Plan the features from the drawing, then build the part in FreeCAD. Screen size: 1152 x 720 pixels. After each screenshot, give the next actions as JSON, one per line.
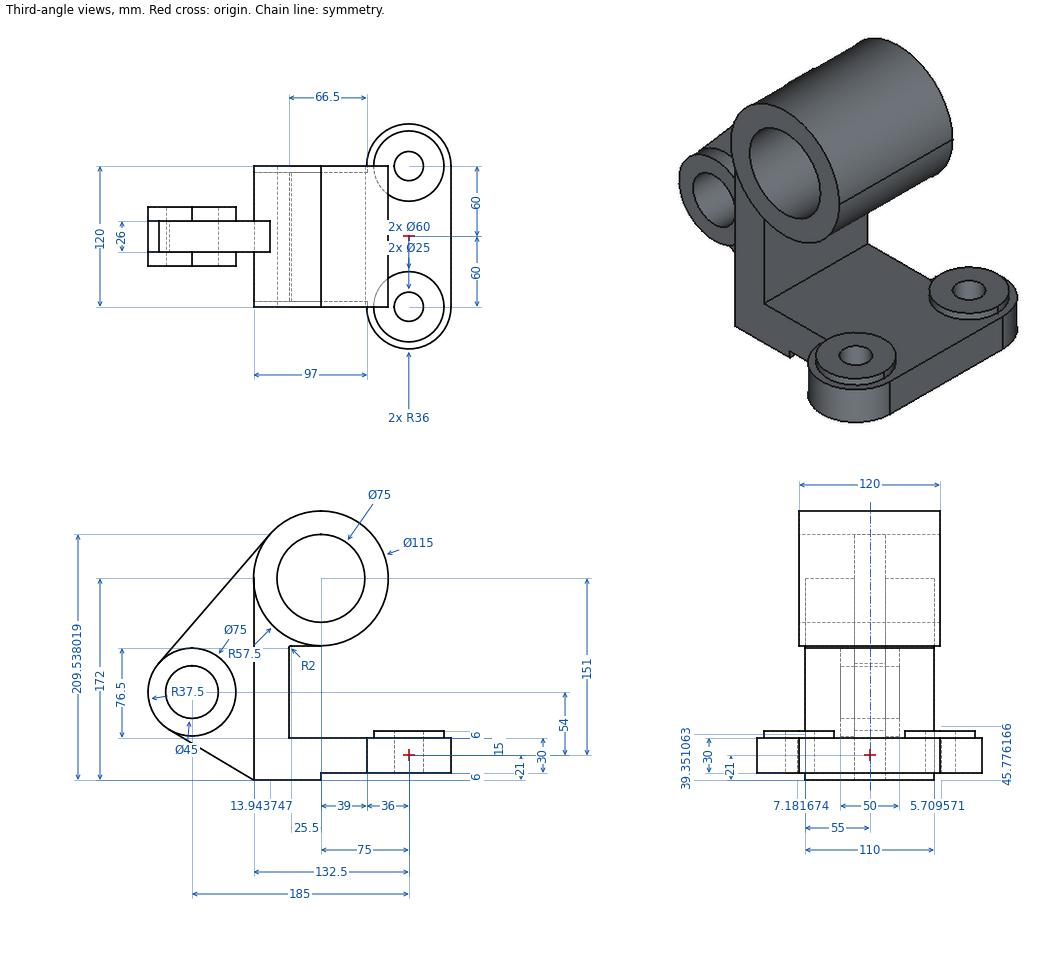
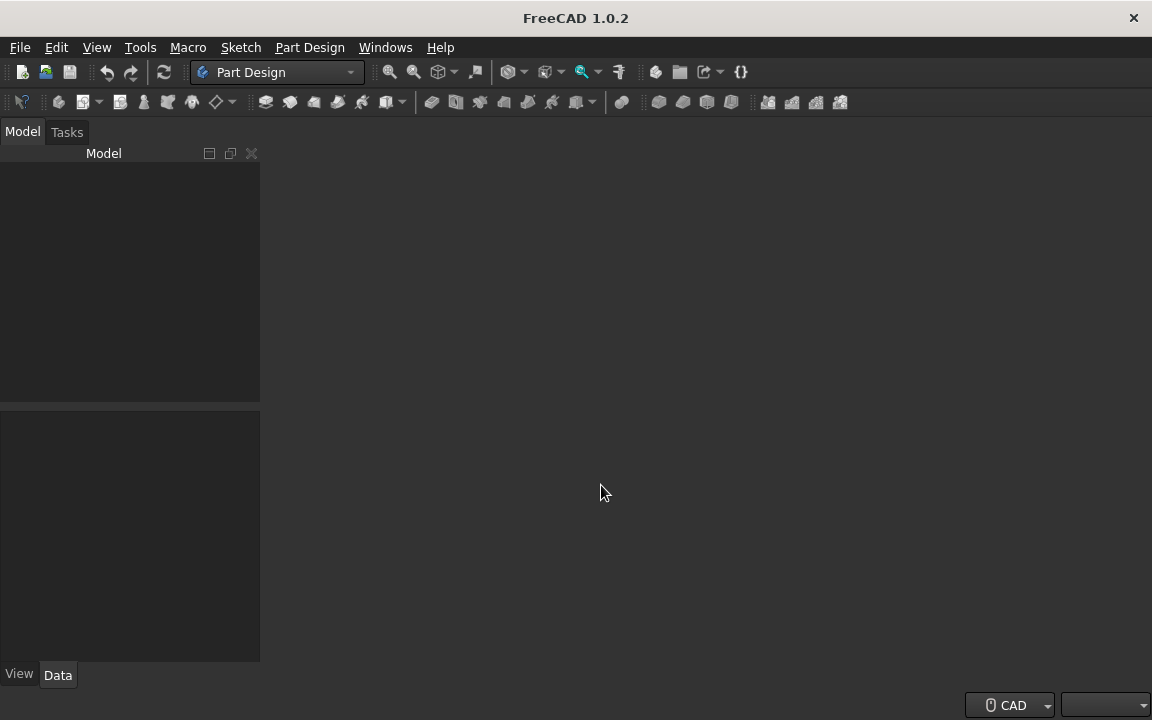
{"action": "left_click", "coordinate": [22, 72]}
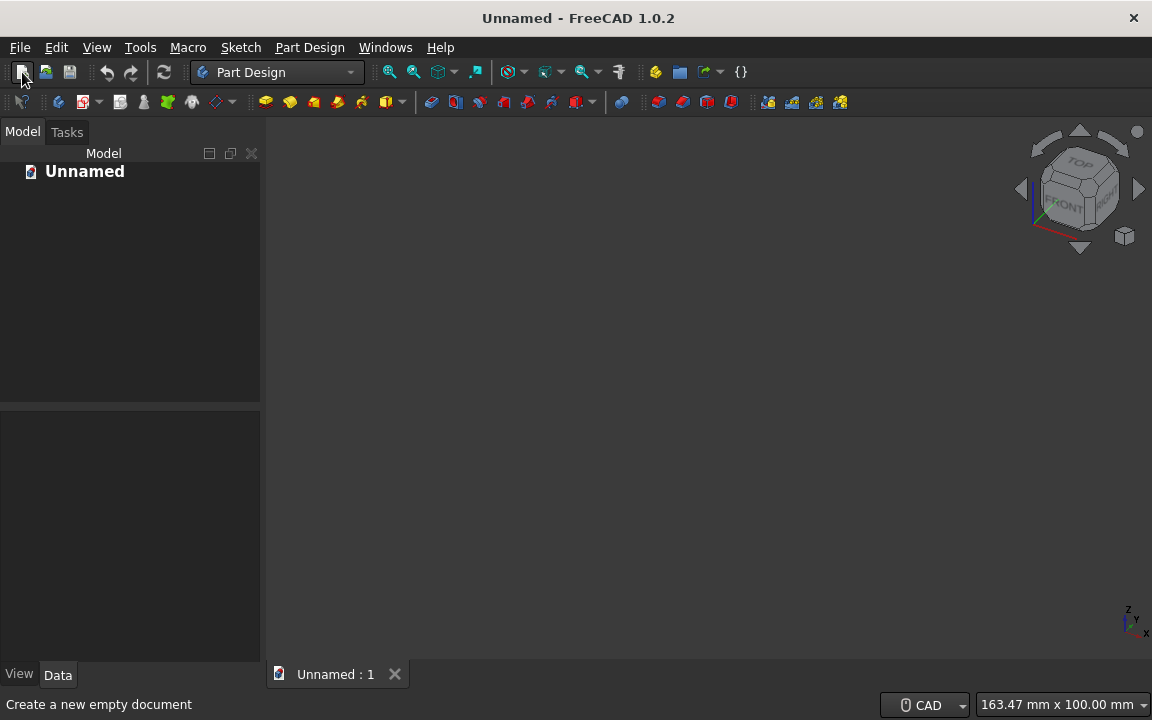
{"action": "left_click", "coordinate": [84, 102]}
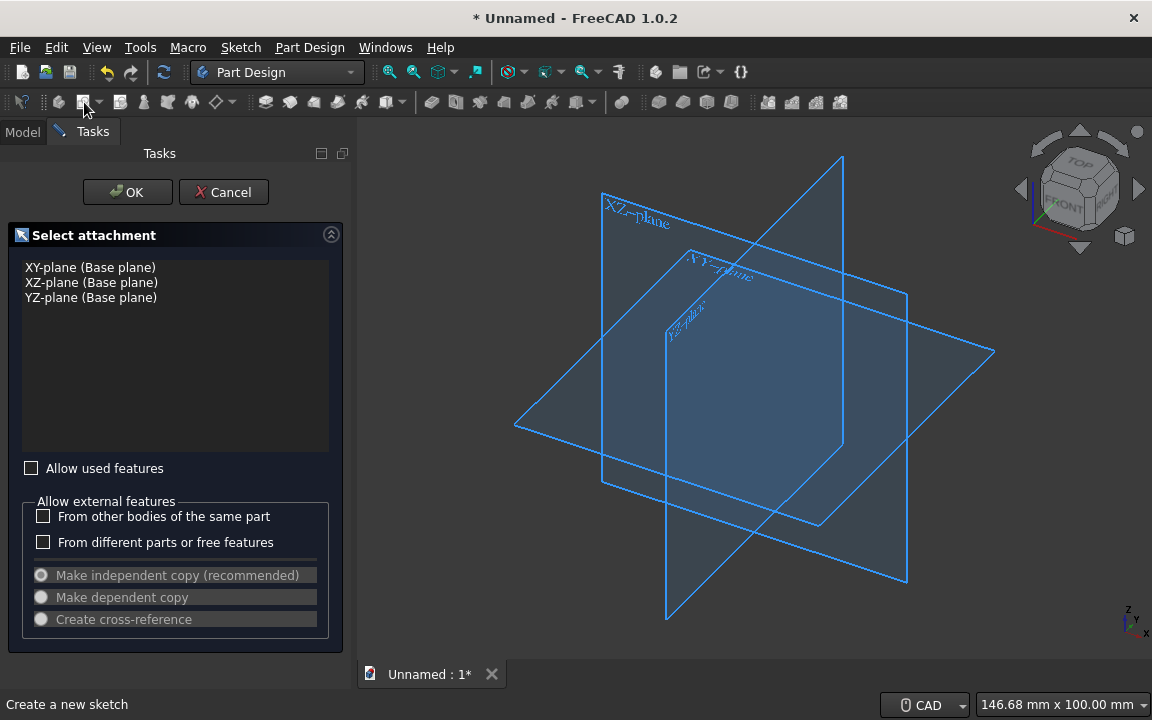
{"action": "left_click", "coordinate": [82, 268]}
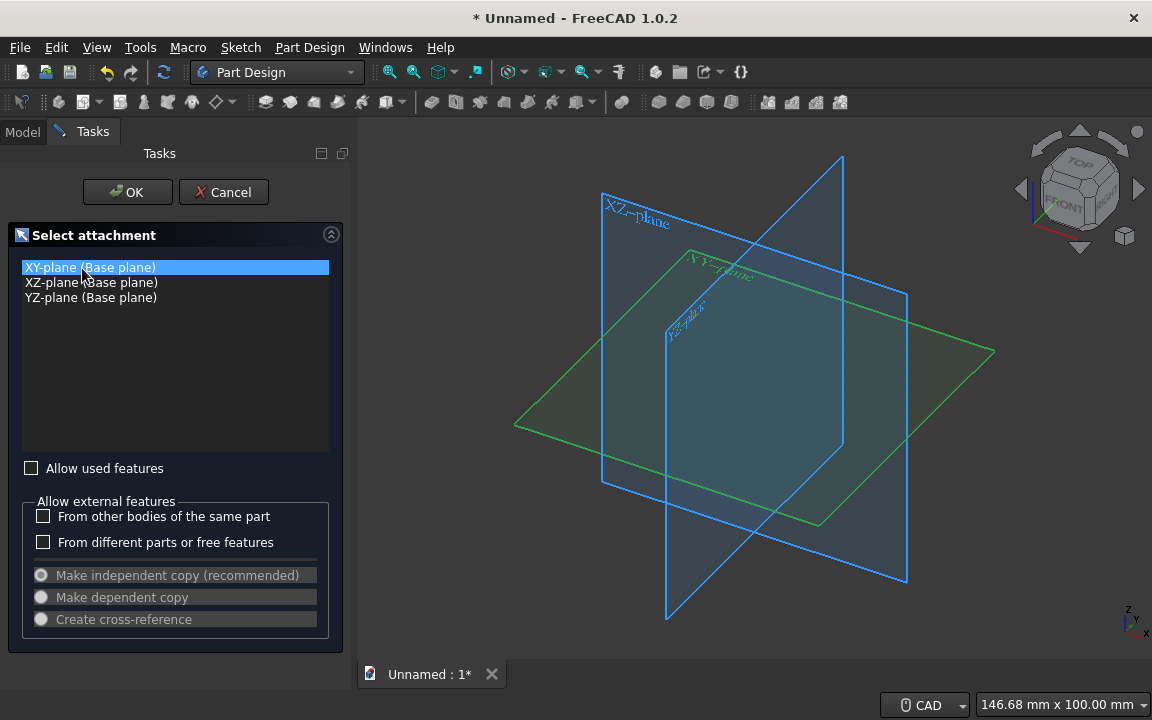
{"action": "left_click", "coordinate": [128, 192]}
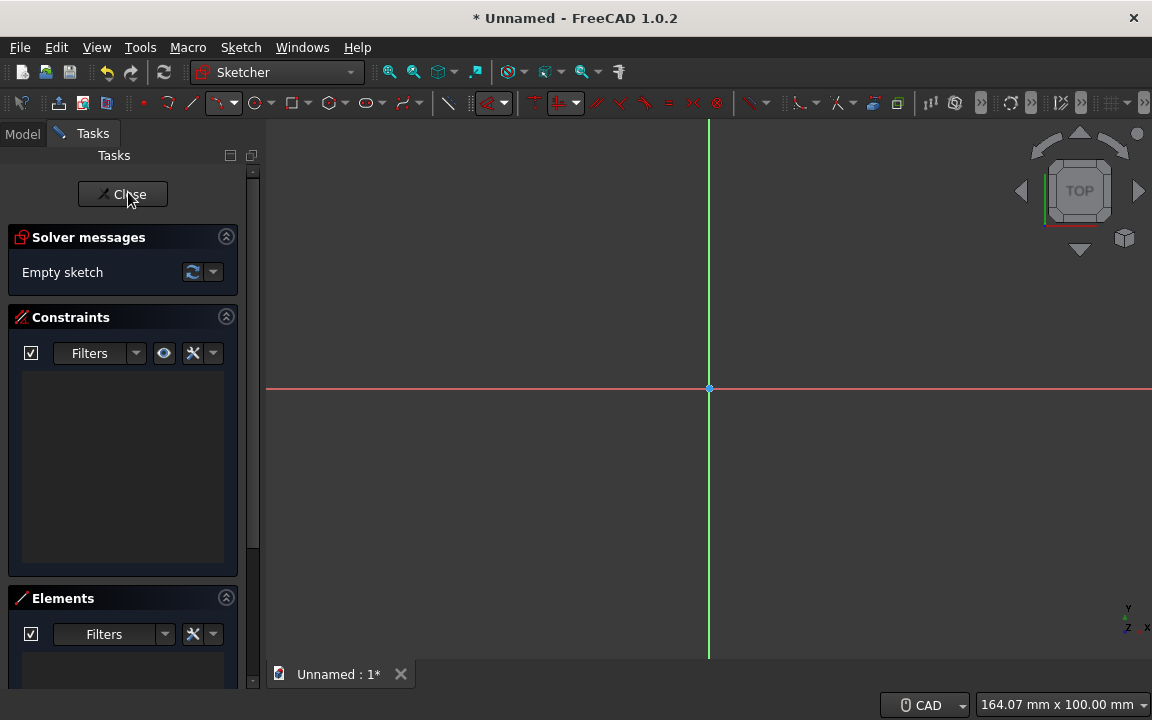
{"action": "scroll", "coordinate": [688, 389], "scroll_direction": "down", "scroll_amount": 6}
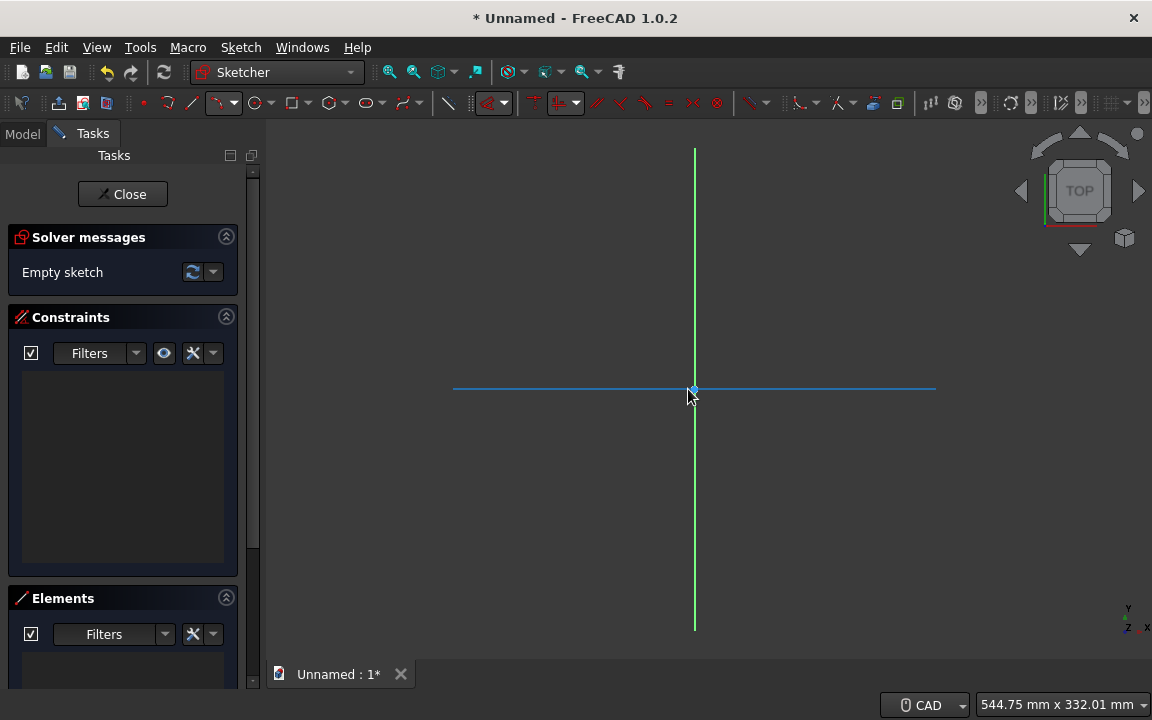
{"action": "left_click", "coordinate": [192, 104]}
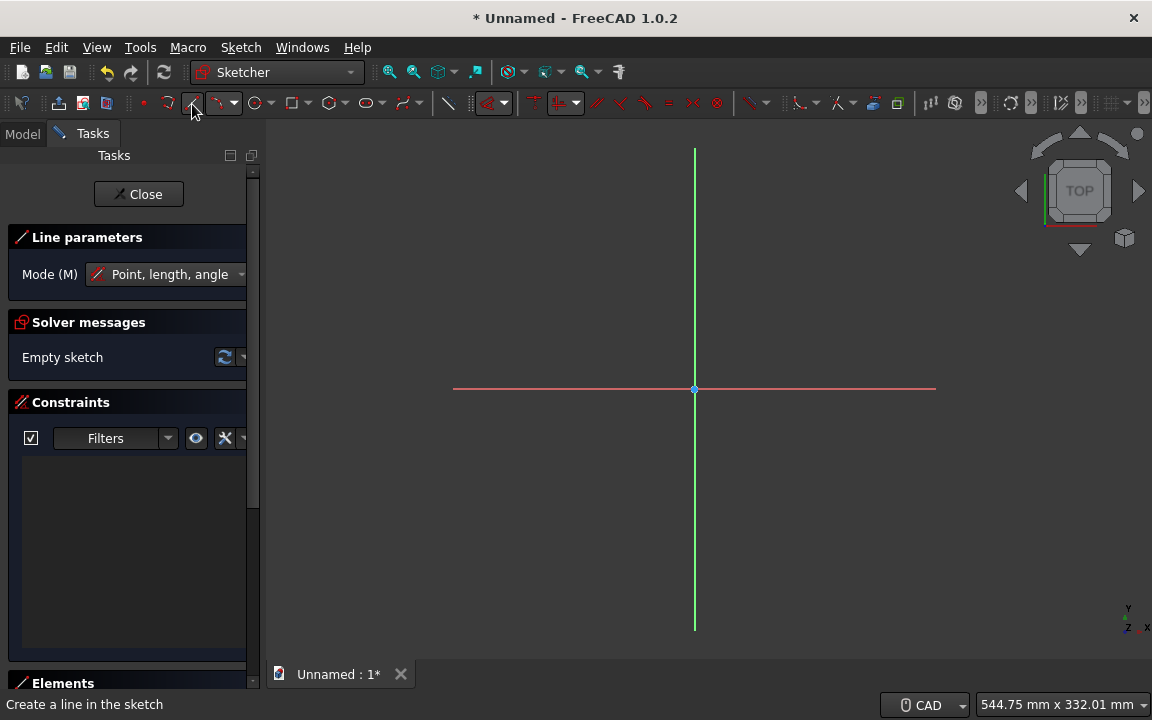
{"action": "left_click", "coordinate": [753, 487]}
{"action": "left_click", "coordinate": [753, 292]}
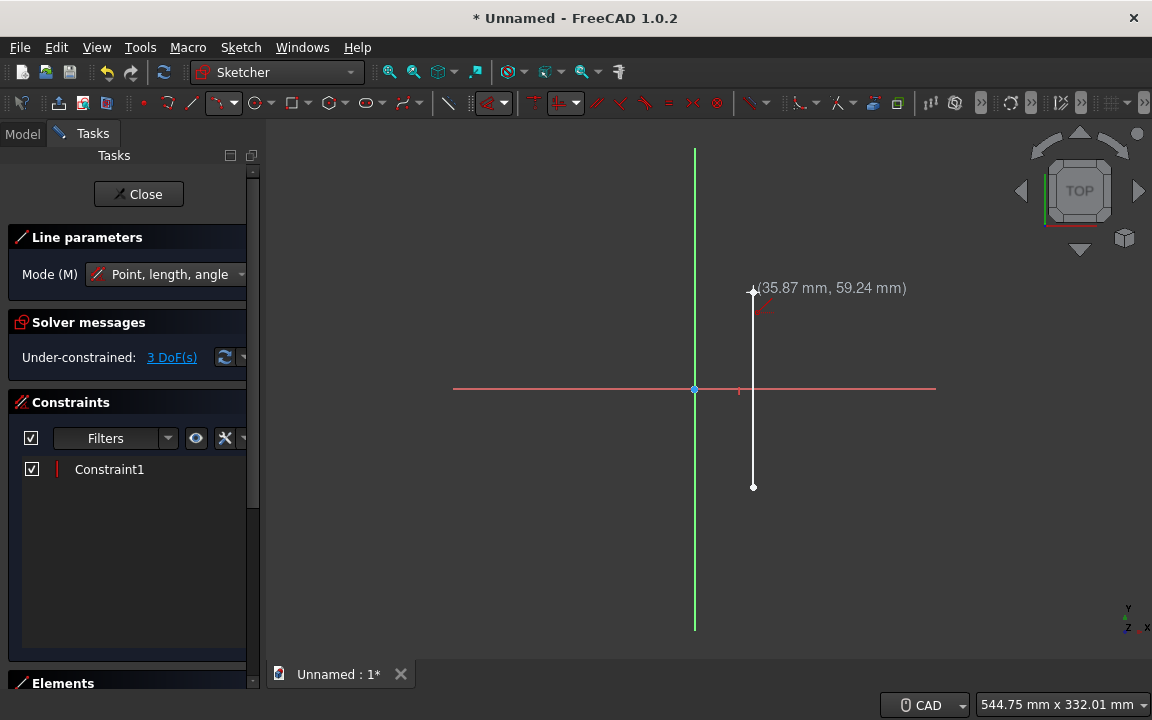
{"action": "key", "text": "g m"}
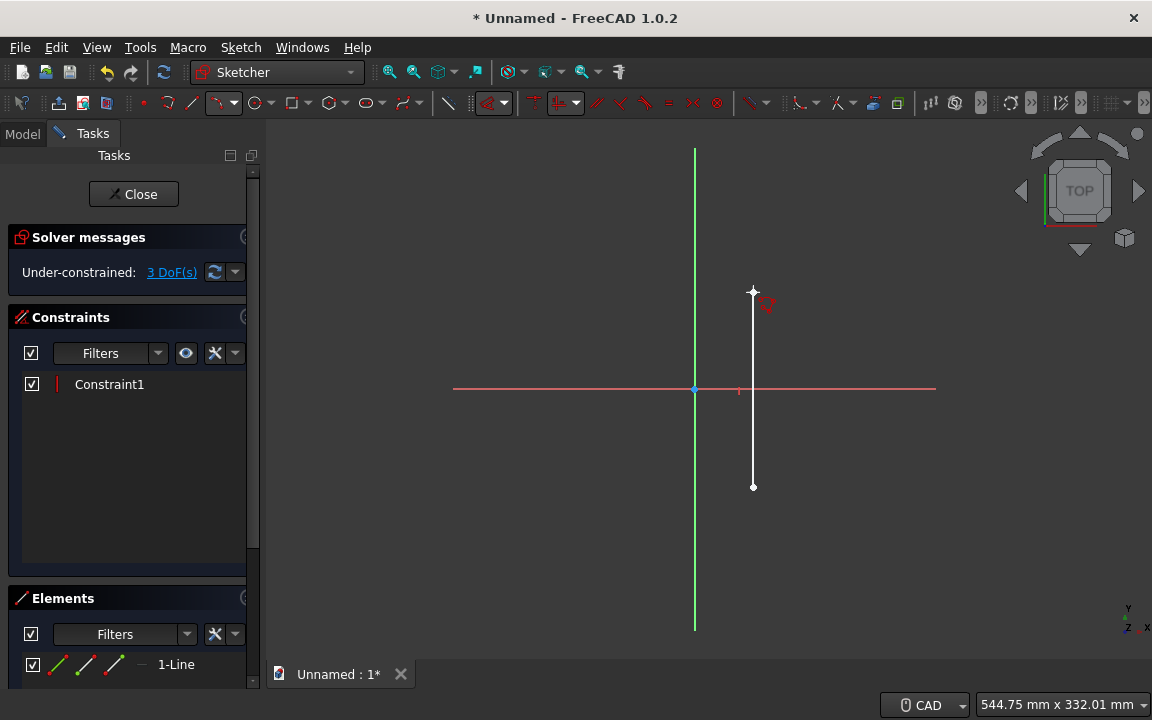
{"action": "left_click", "coordinate": [636, 292]}
{"action": "left_click", "coordinate": [528, 292]}
{"action": "left_click", "coordinate": [528, 487]}
{"action": "left_click", "coordinate": [636, 487]}
{"action": "right_click", "coordinate": [636, 487]}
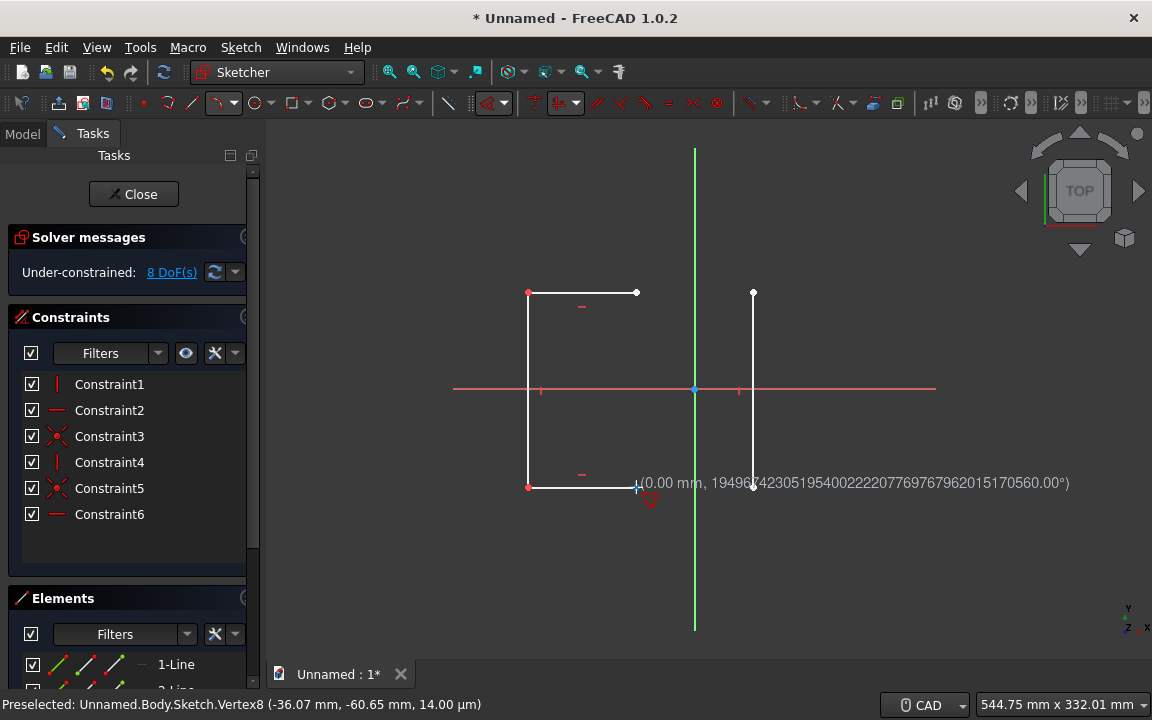
{"action": "key", "text": "g 3 a"}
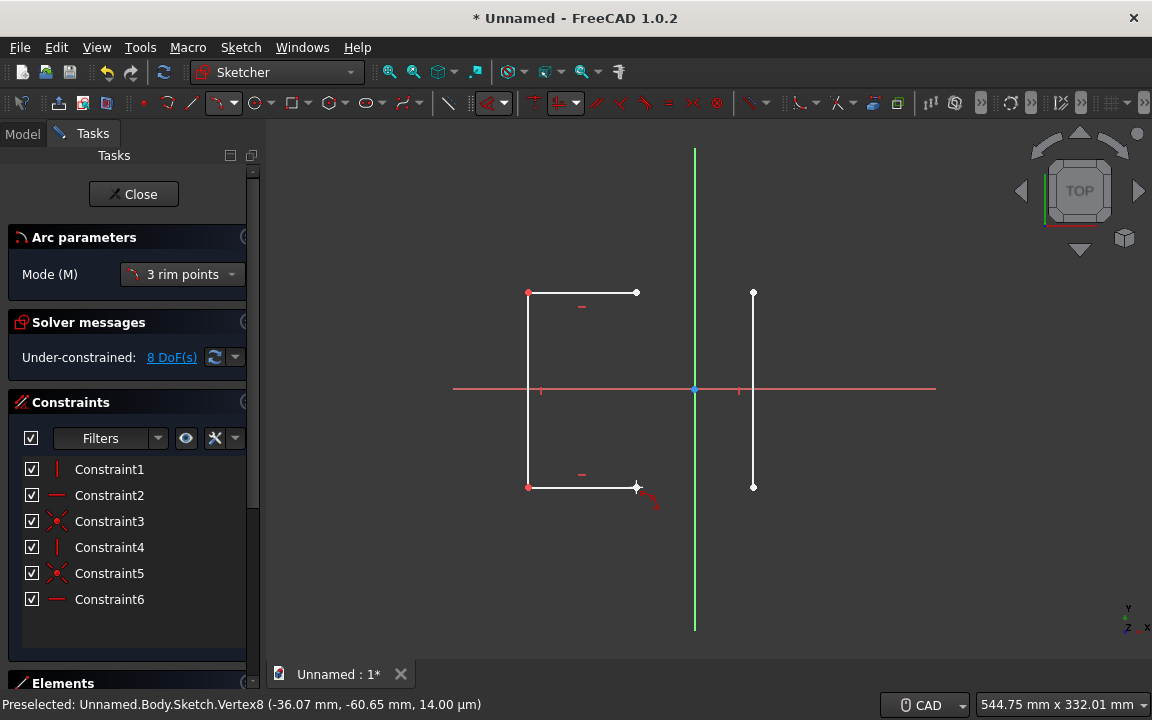
{"action": "left_click", "coordinate": [753, 293]}
{"action": "left_click", "coordinate": [636, 293]}
{"action": "left_click", "coordinate": [713, 236]}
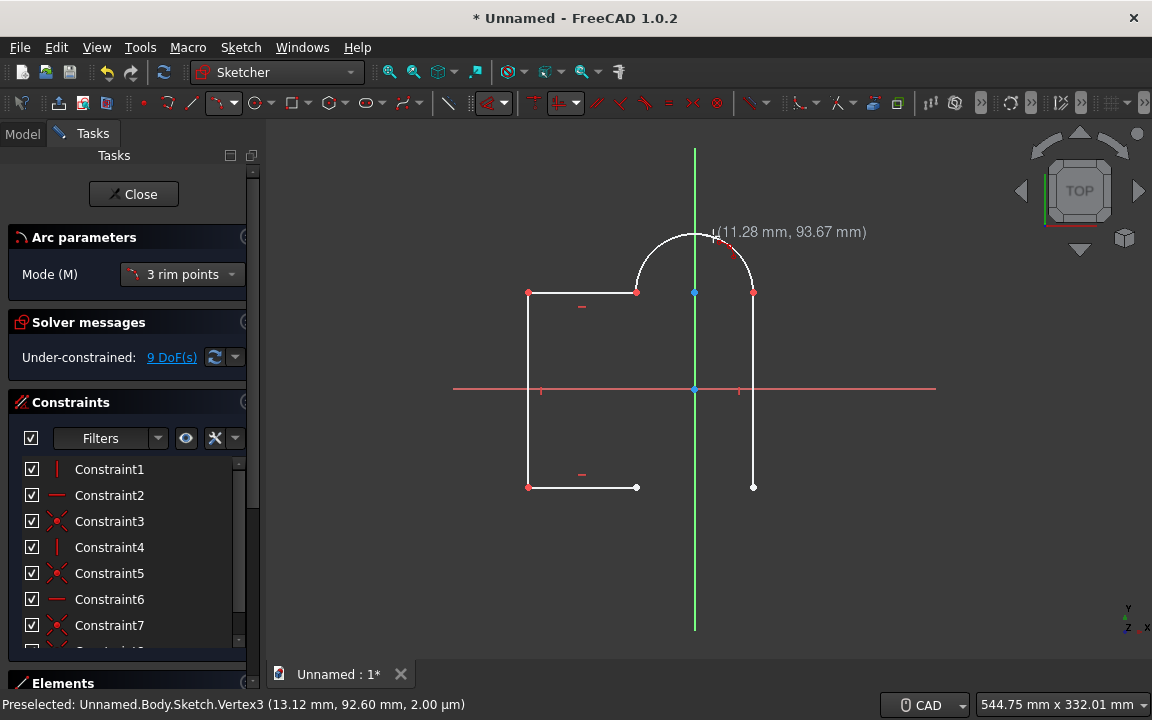
{"action": "left_click", "coordinate": [636, 488]}
{"action": "left_click", "coordinate": [753, 488]}
{"action": "left_click", "coordinate": [677, 543]}